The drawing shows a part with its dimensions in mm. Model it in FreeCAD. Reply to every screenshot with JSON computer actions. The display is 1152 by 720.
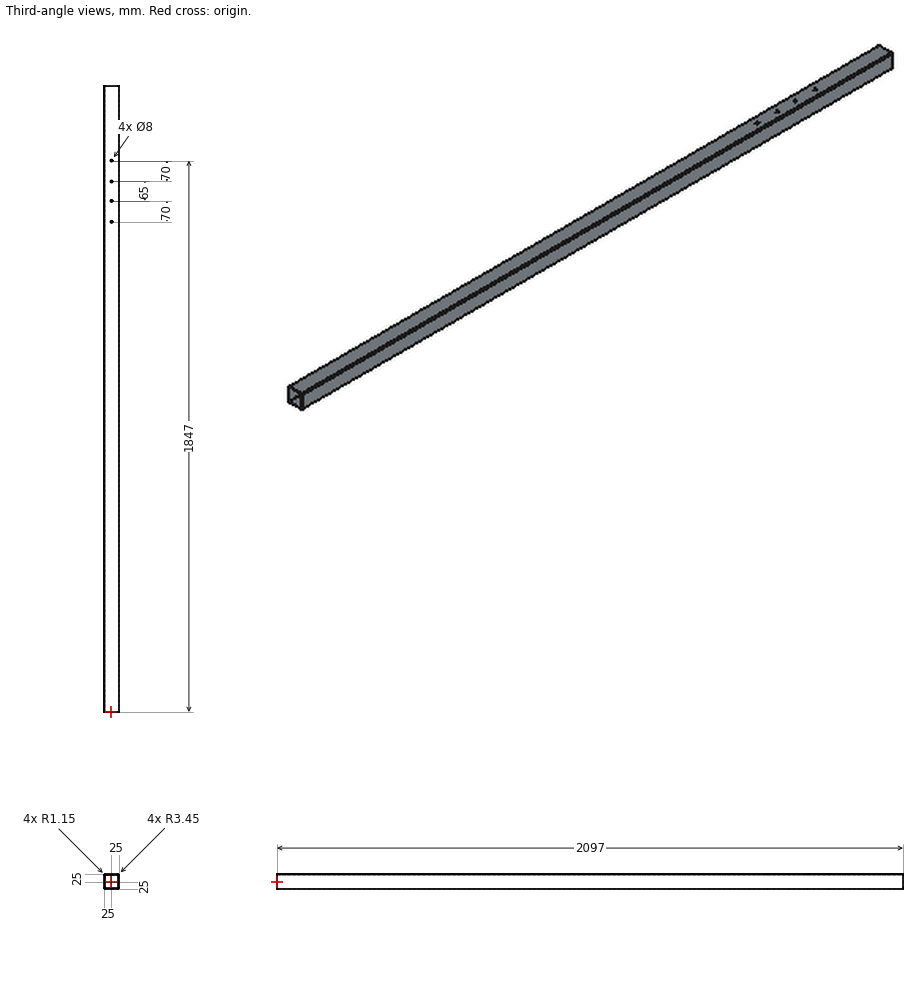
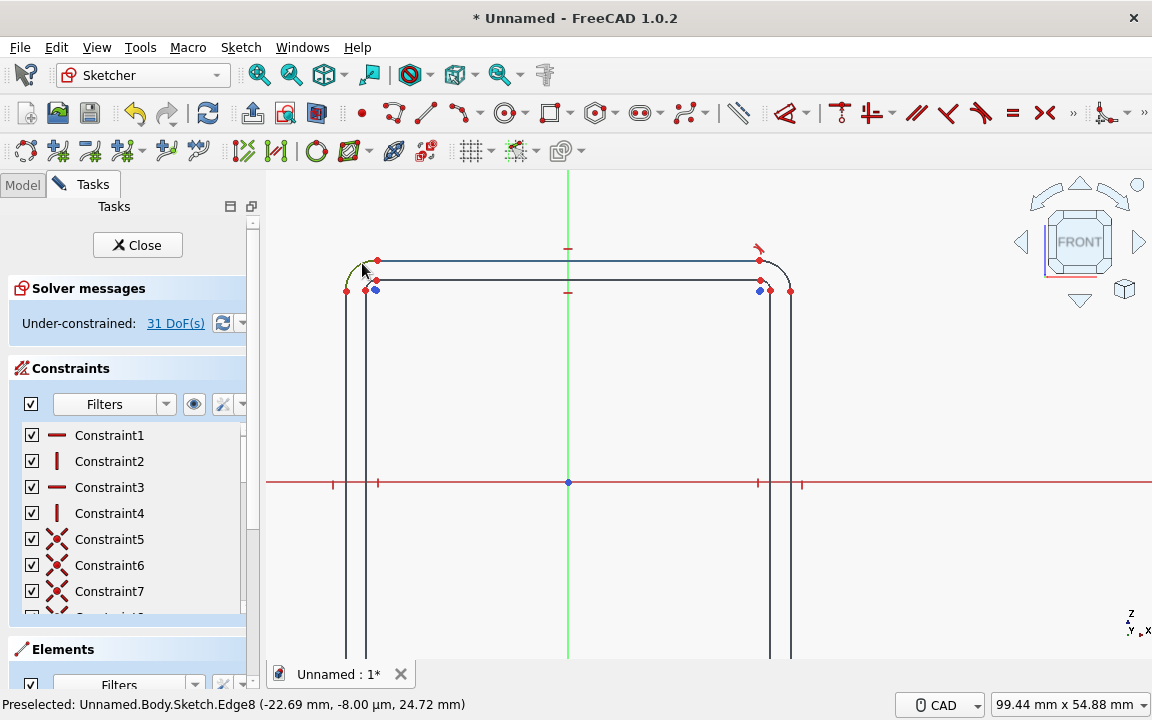
{"action": "left_click", "coordinate": [982, 114]}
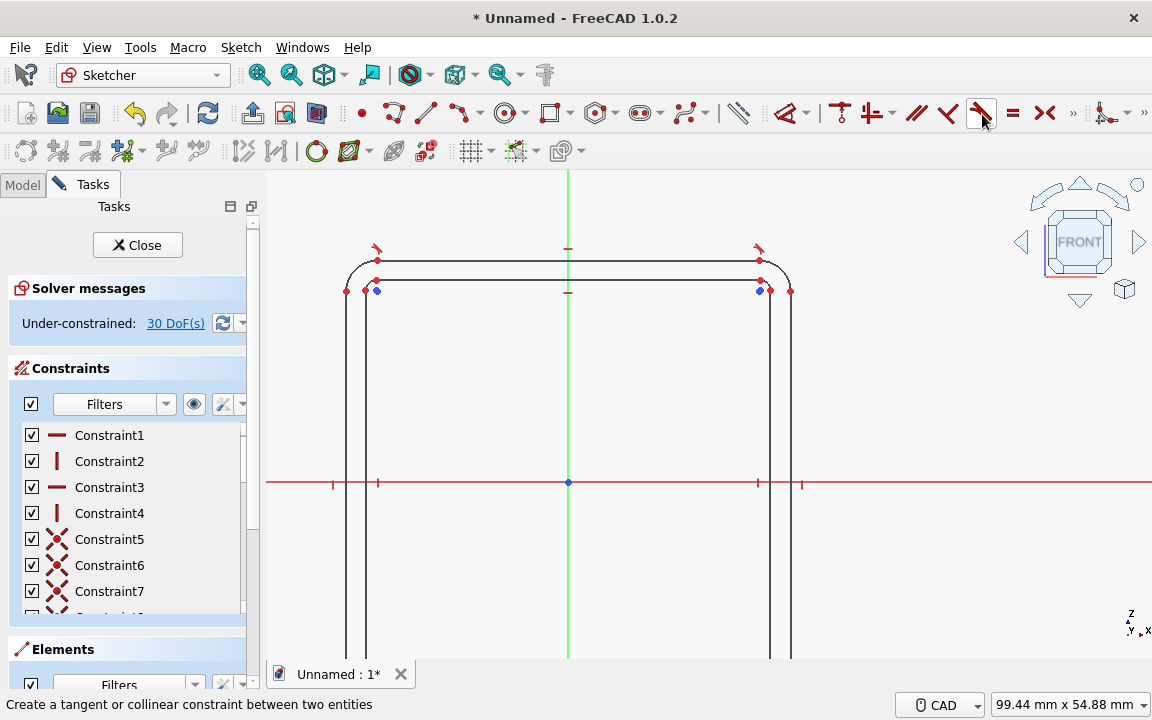
{"action": "left_click", "coordinate": [791, 407]}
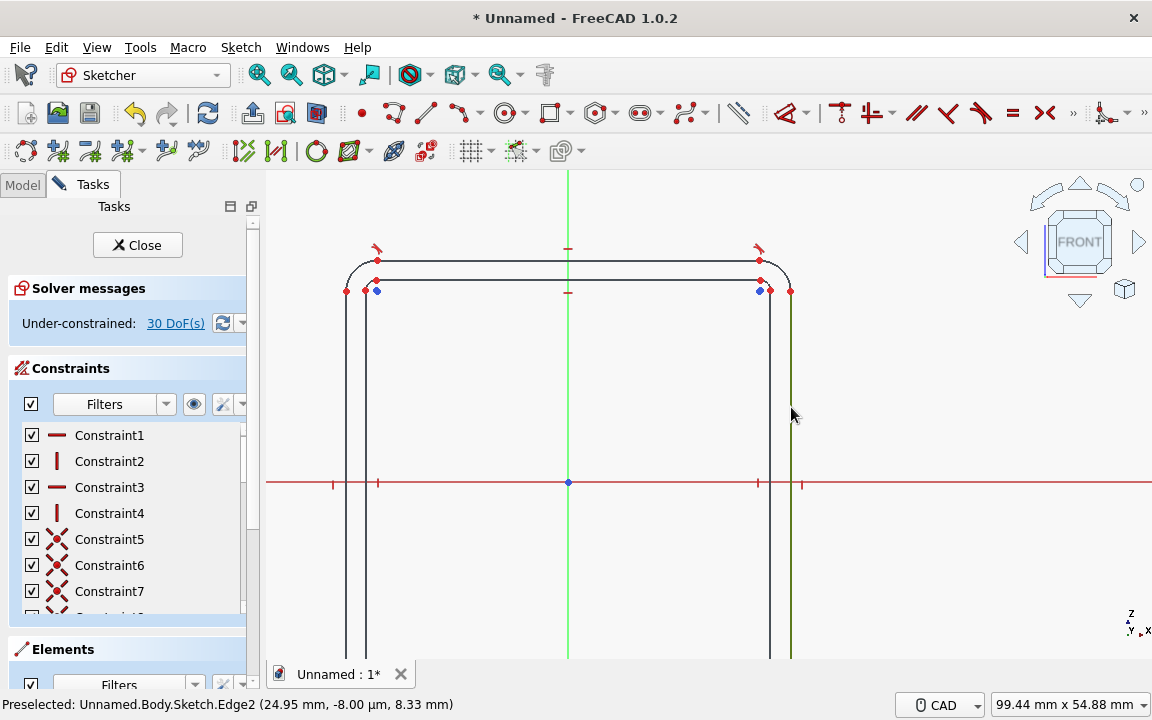
{"action": "left_click", "coordinate": [787, 278]}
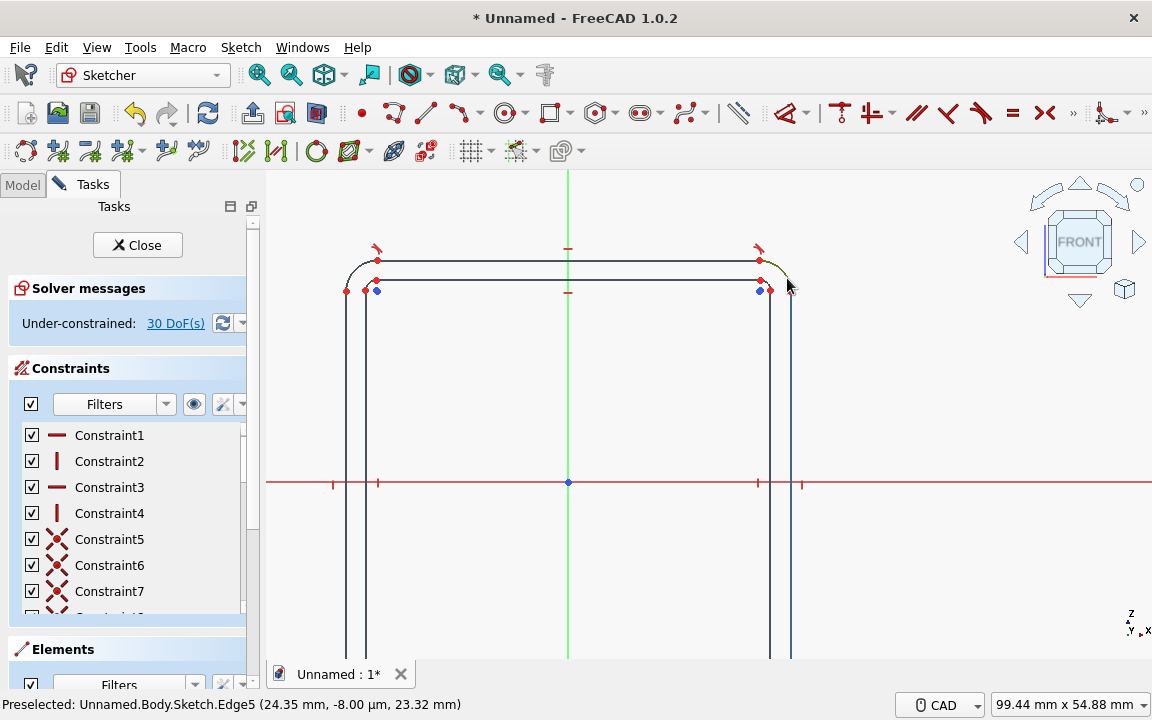
{"action": "left_click", "coordinate": [982, 114]}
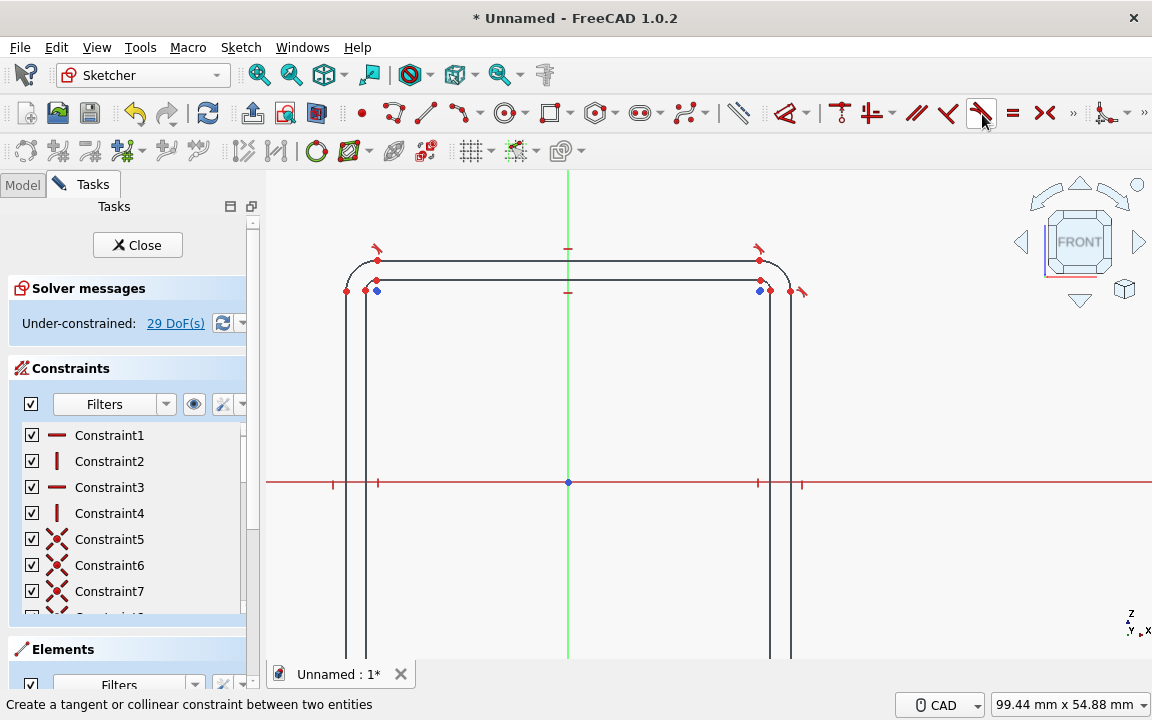
{"action": "left_click", "coordinate": [791, 407]}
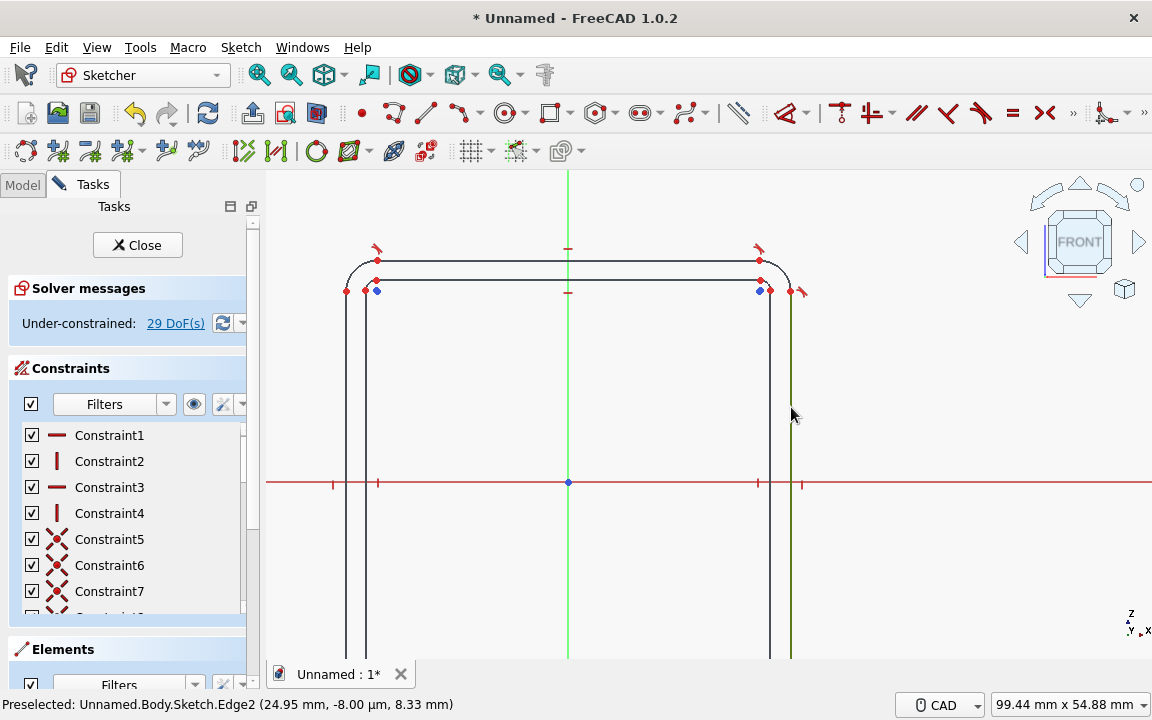
{"action": "scroll", "coordinate": [787, 277], "scroll_direction": "down", "scroll_amount": 2}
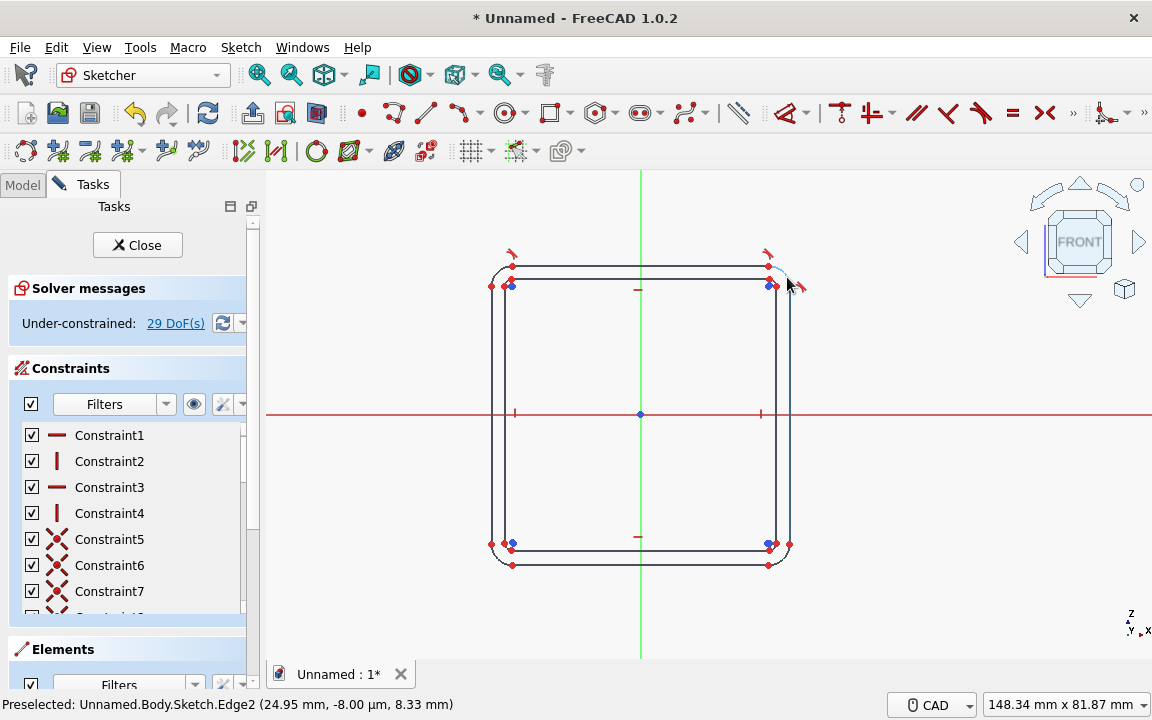
{"action": "scroll", "coordinate": [778, 563], "scroll_direction": "up", "scroll_amount": 2}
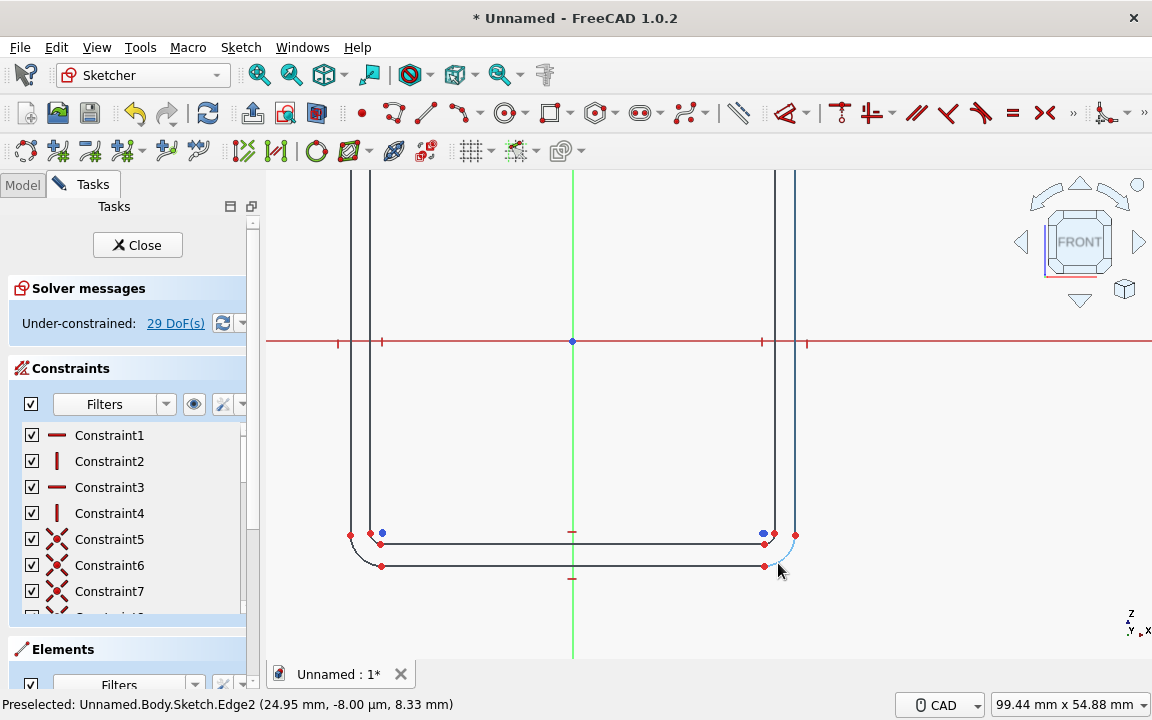
{"action": "left_click", "coordinate": [778, 563]}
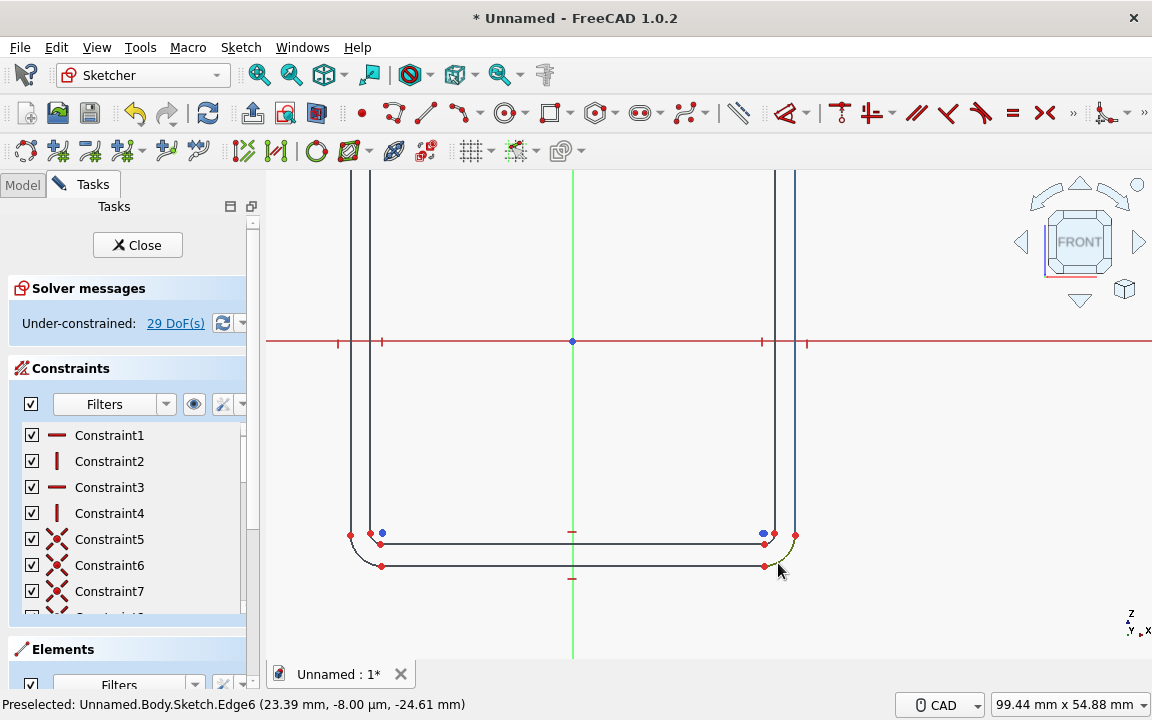
{"action": "left_click", "coordinate": [982, 114]}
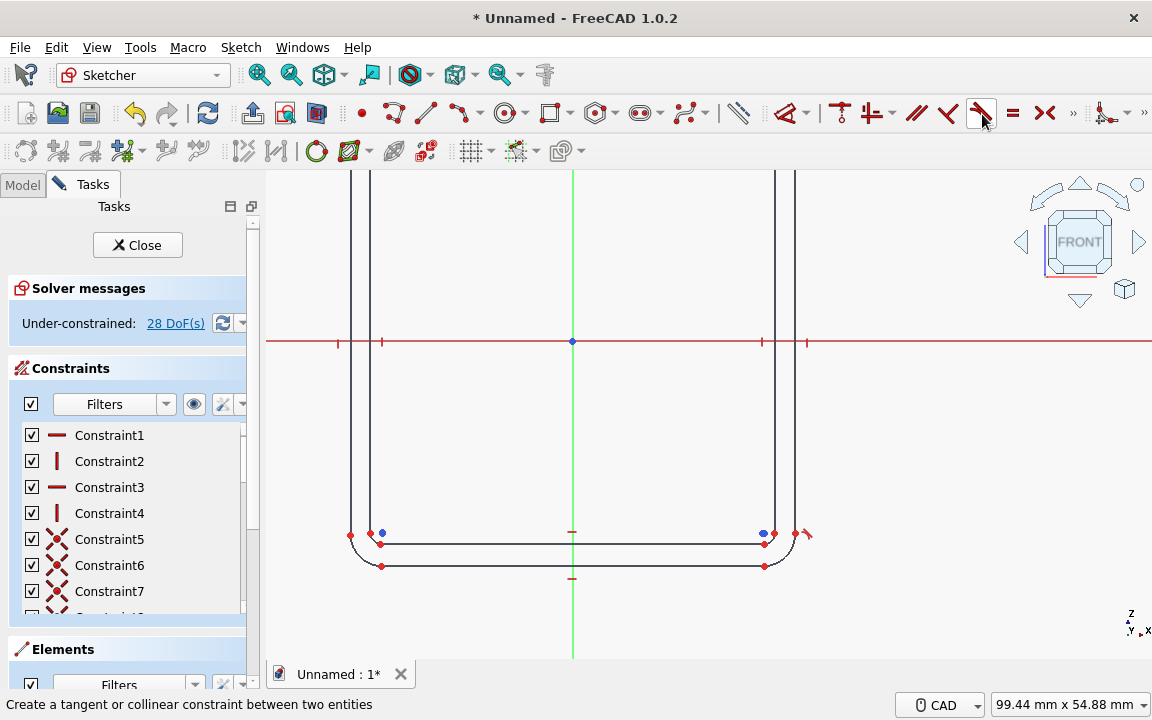
{"action": "left_click", "coordinate": [649, 566]}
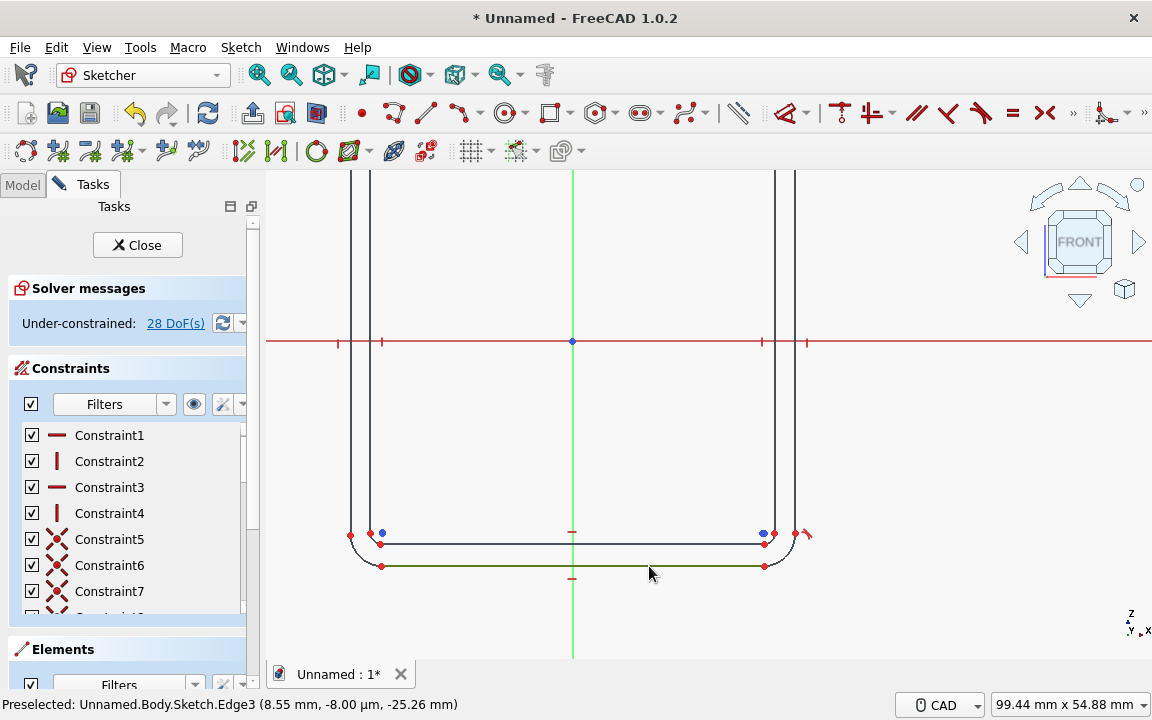
{"action": "left_click", "coordinate": [778, 562]}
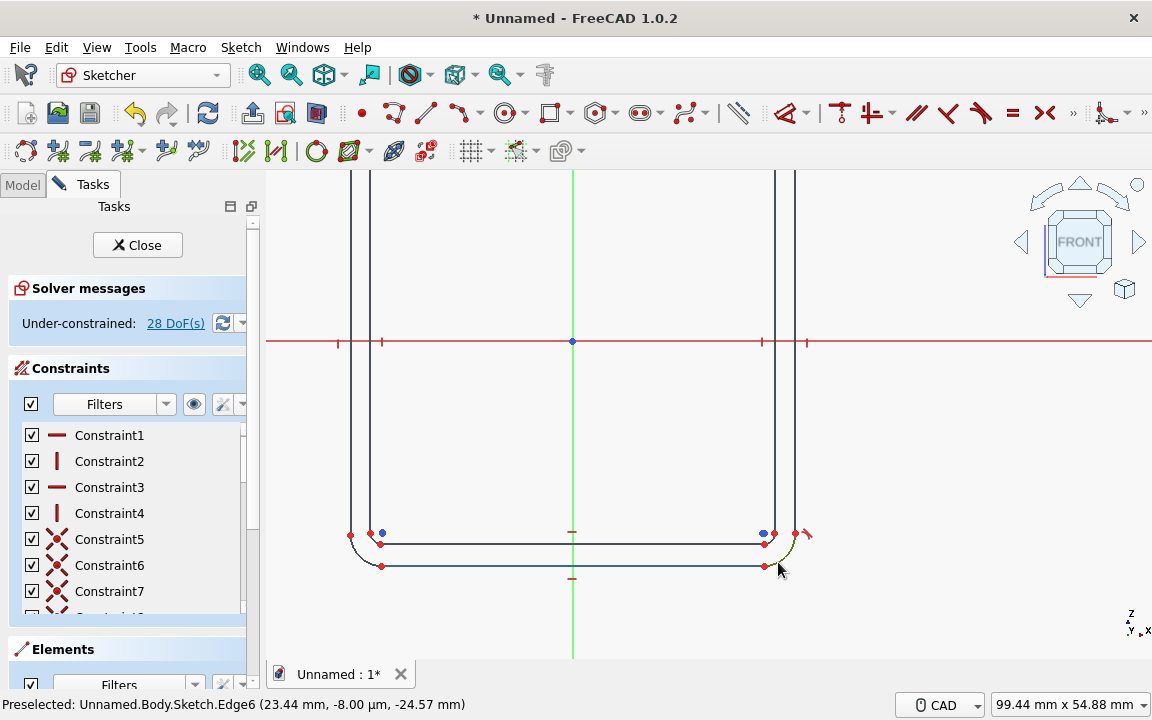
{"action": "left_click", "coordinate": [982, 114]}